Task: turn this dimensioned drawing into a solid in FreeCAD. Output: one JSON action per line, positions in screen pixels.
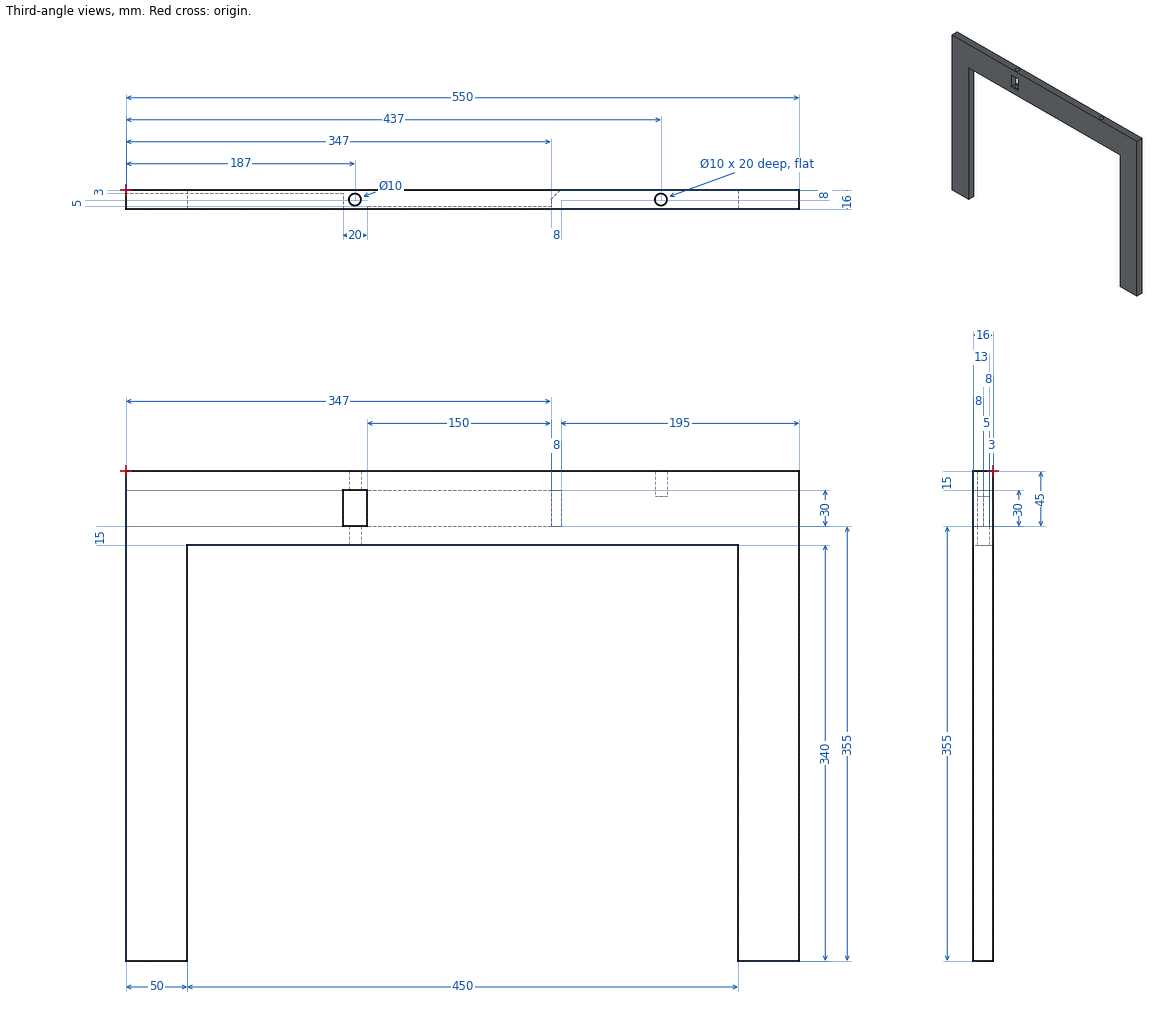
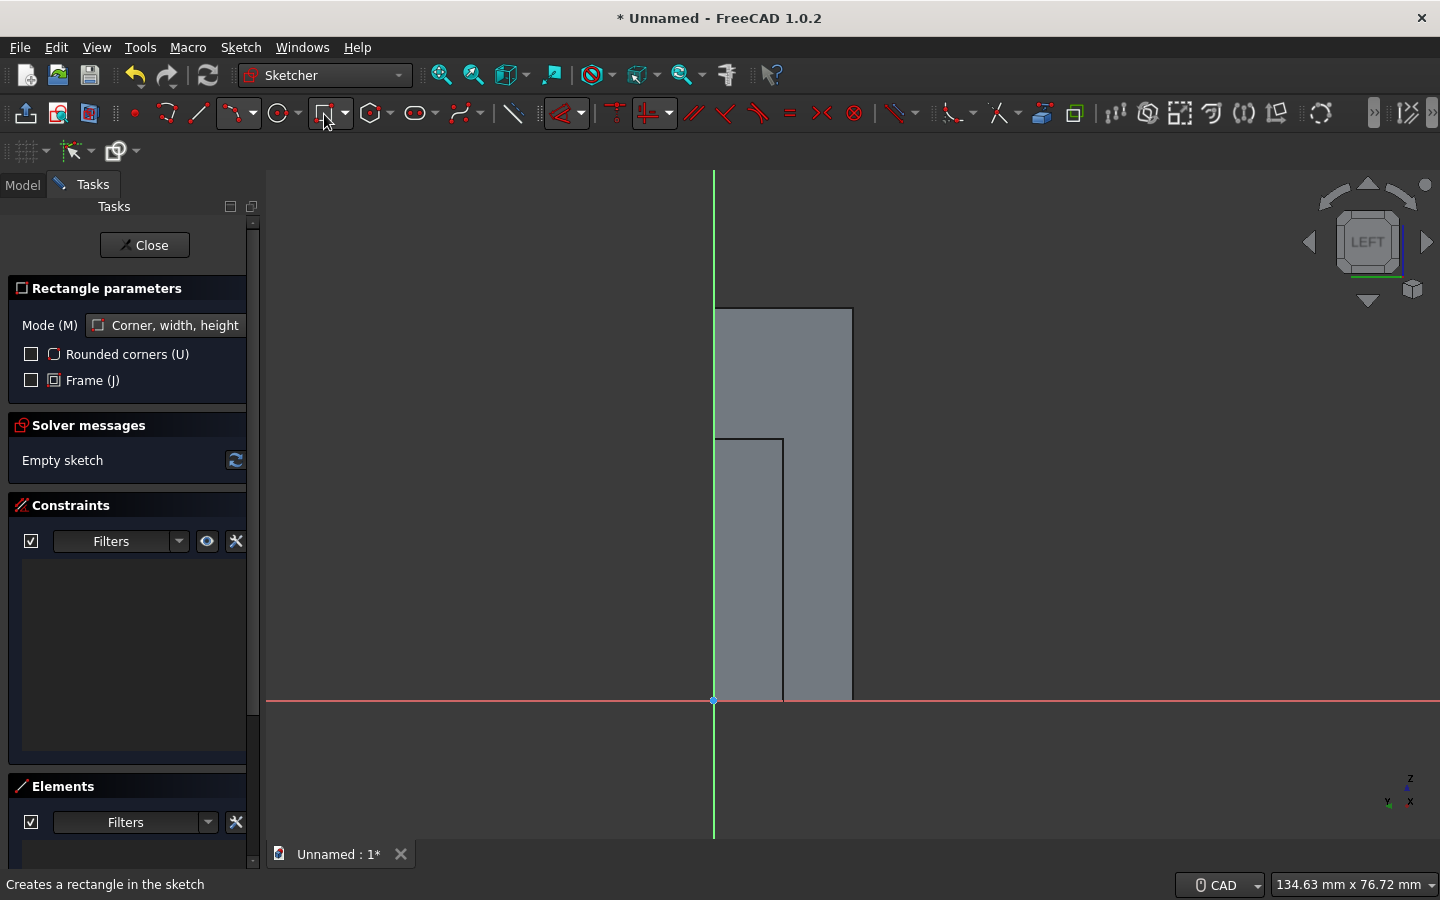
{"action": "left_click", "coordinate": [714, 701]}
{"action": "left_click", "coordinate": [853, 308]}
{"action": "key", "text": "Escape"}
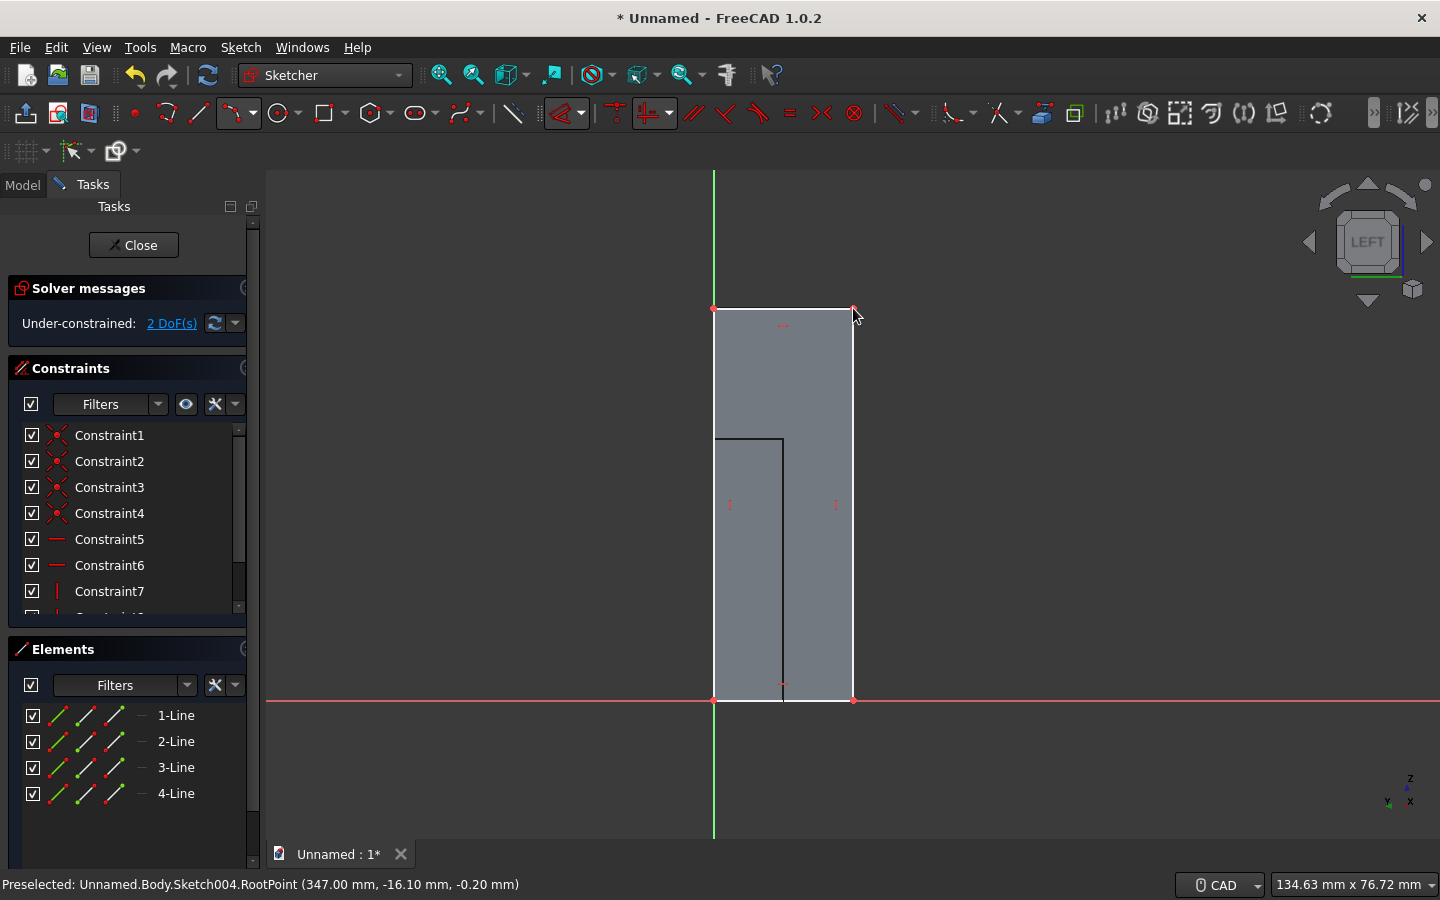
{"action": "left_click", "coordinate": [755, 701]}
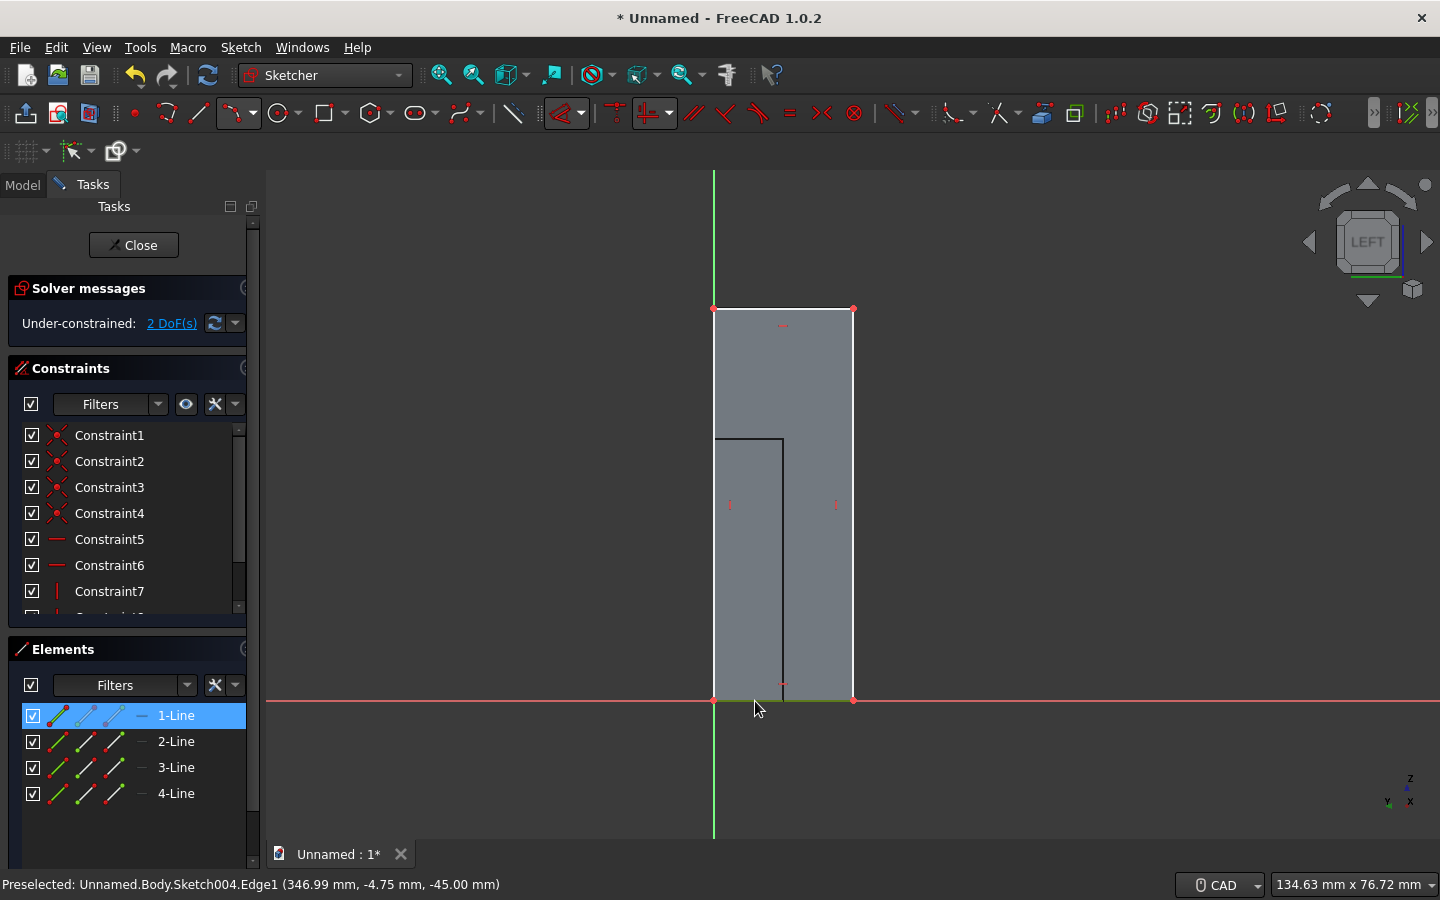
{"action": "left_click", "coordinate": [584, 114]}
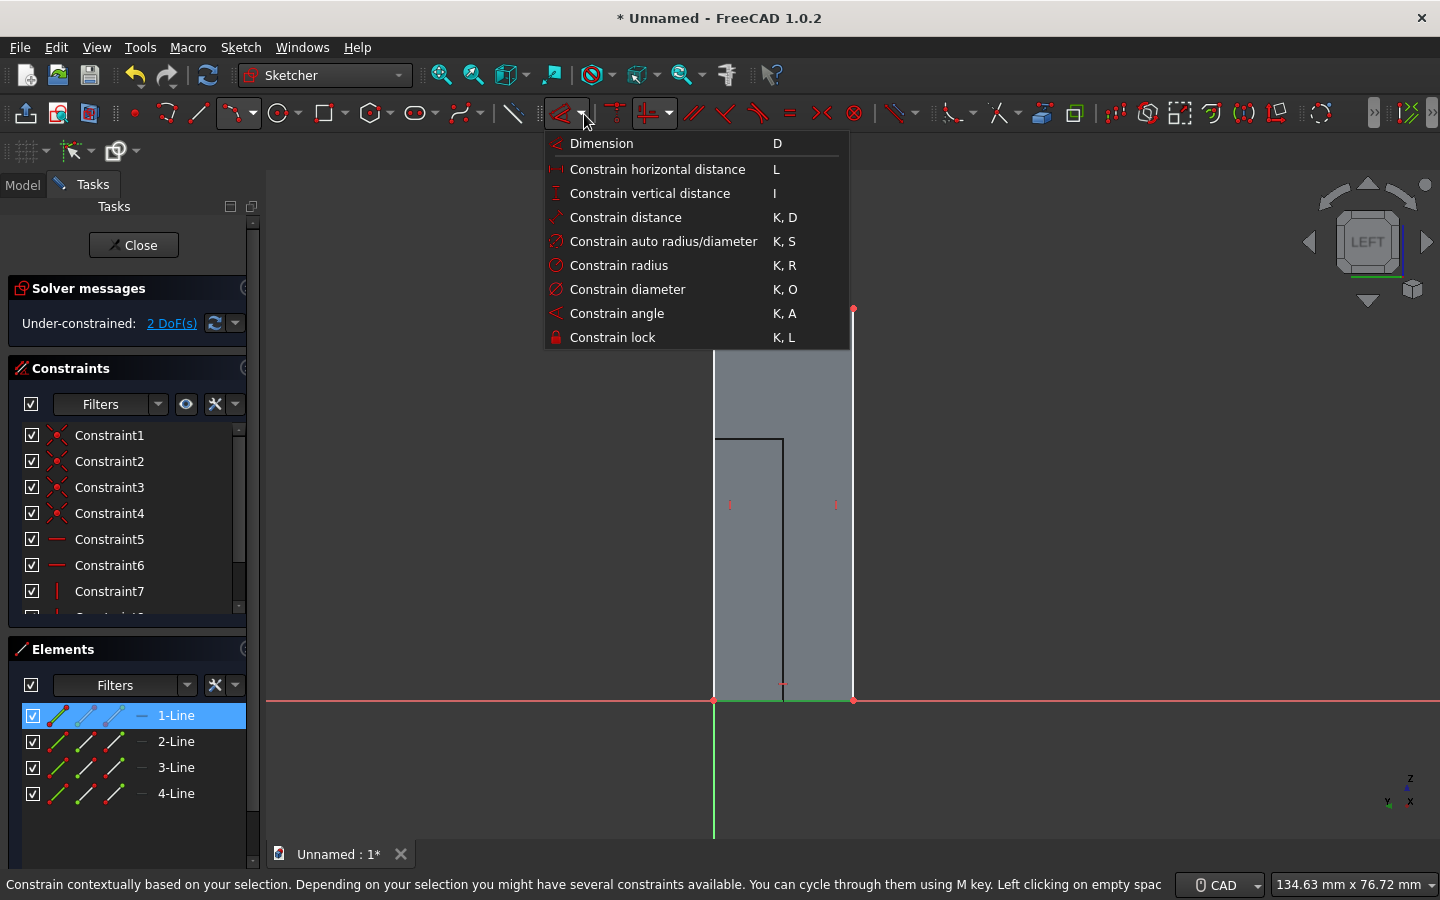
{"action": "left_click", "coordinate": [697, 169]}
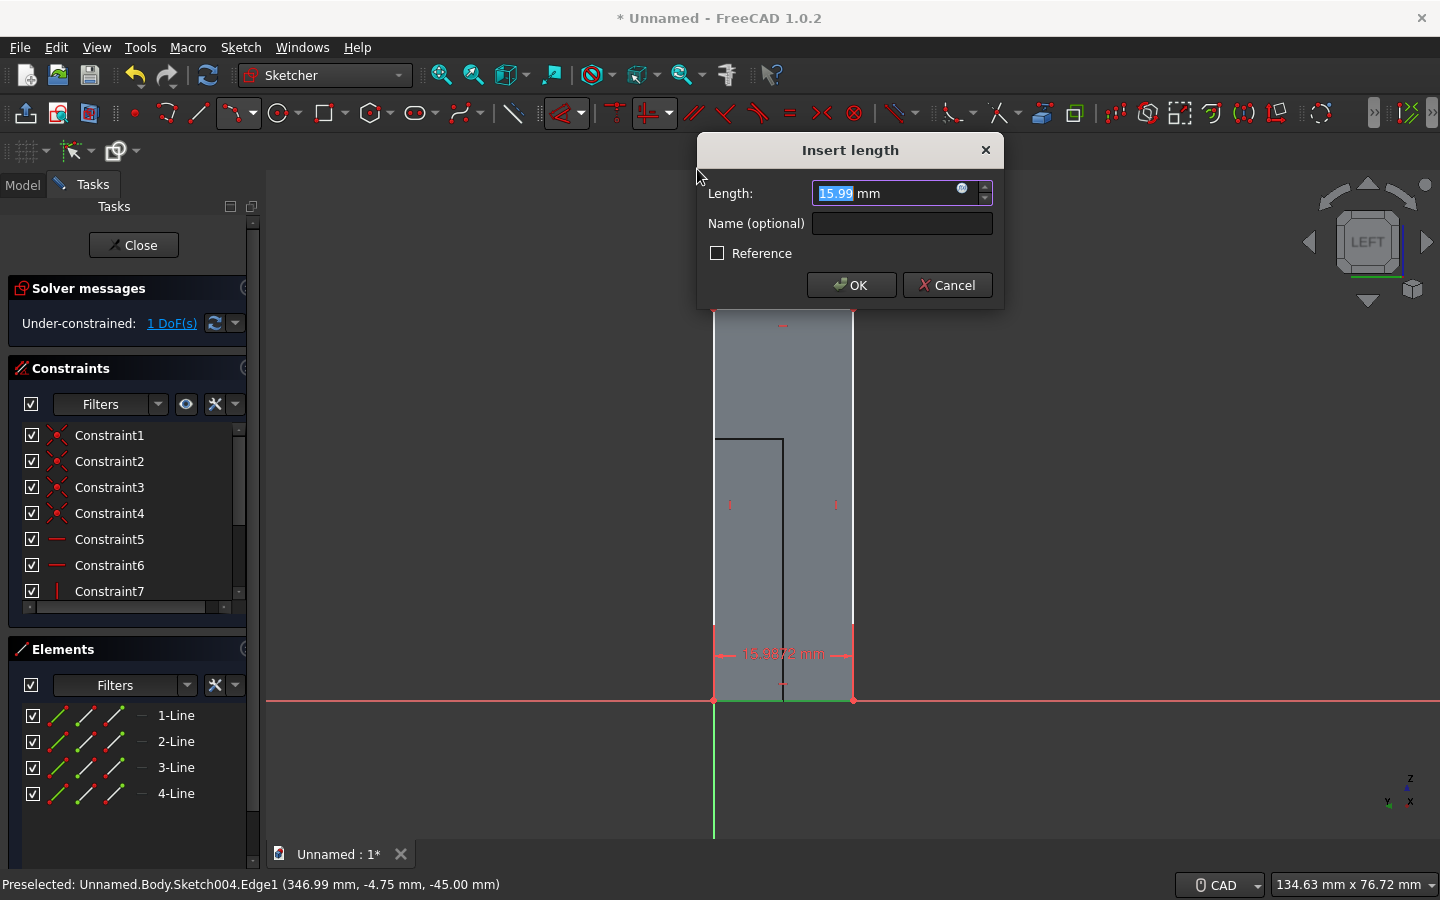
{"action": "type", "text": "16"}
{"action": "key", "text": "Return"}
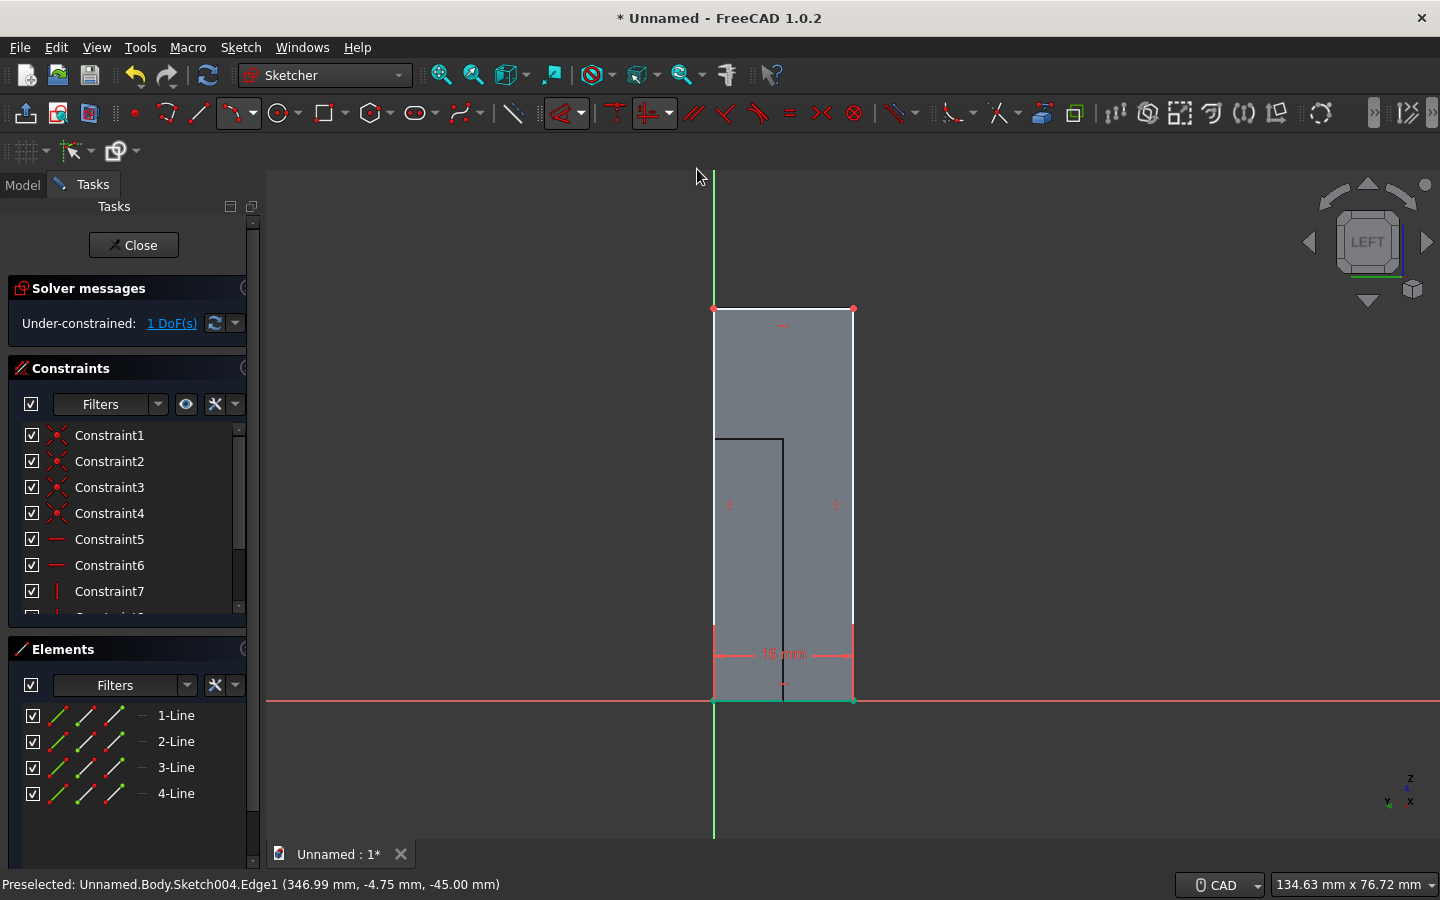
{"action": "left_click", "coordinate": [853, 583]}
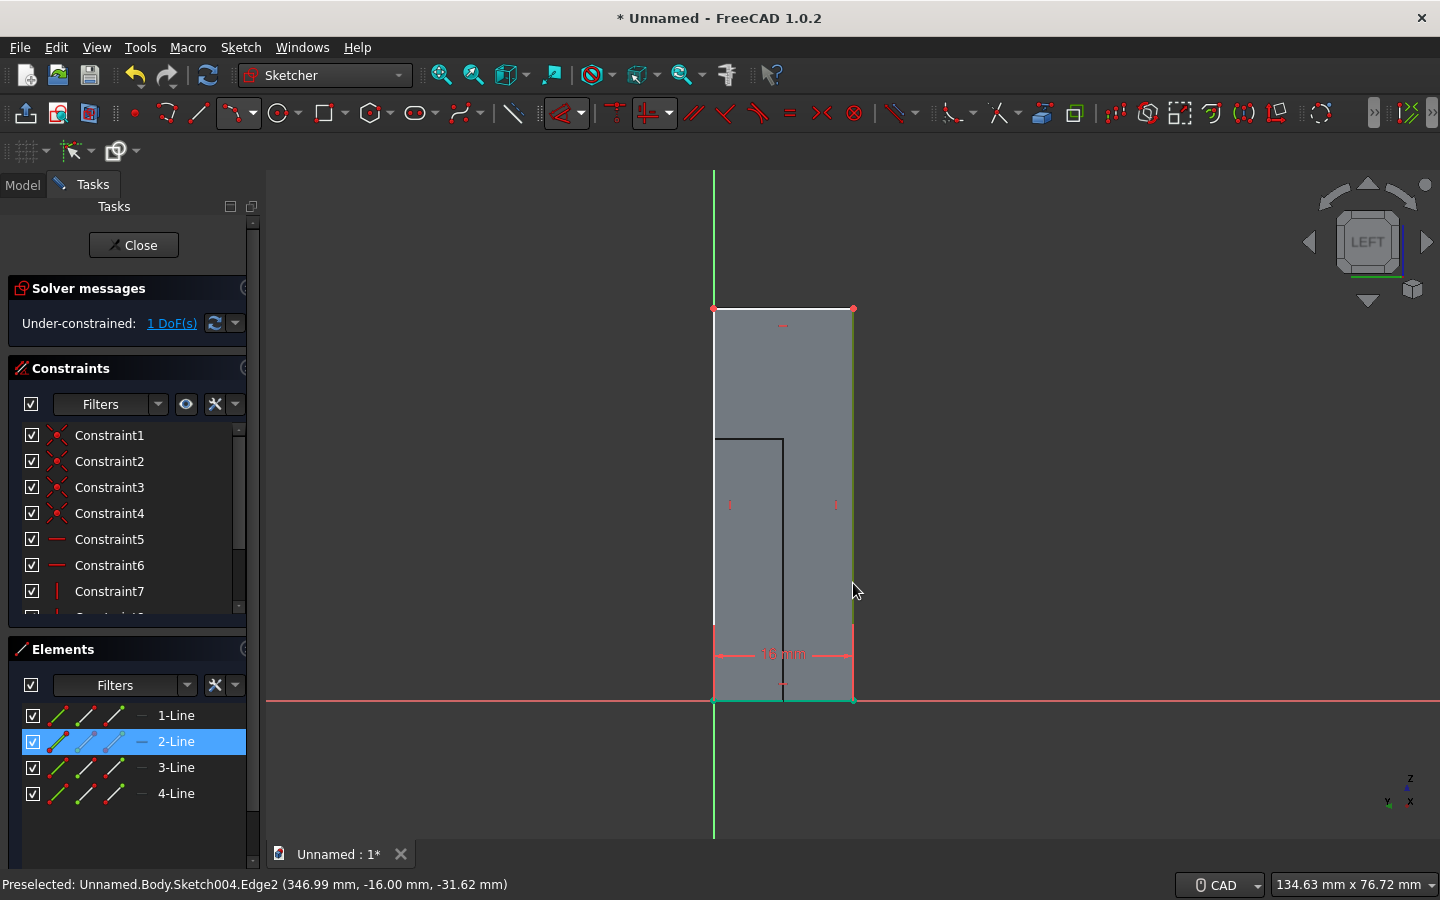
{"action": "left_click", "coordinate": [584, 114]}